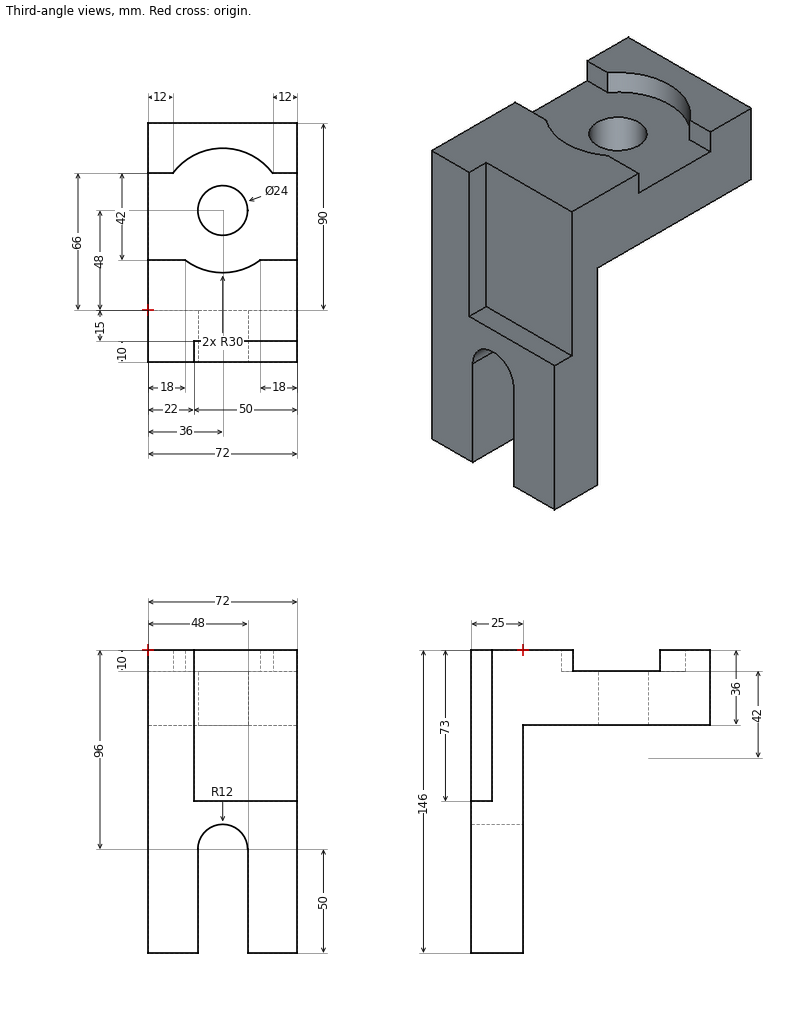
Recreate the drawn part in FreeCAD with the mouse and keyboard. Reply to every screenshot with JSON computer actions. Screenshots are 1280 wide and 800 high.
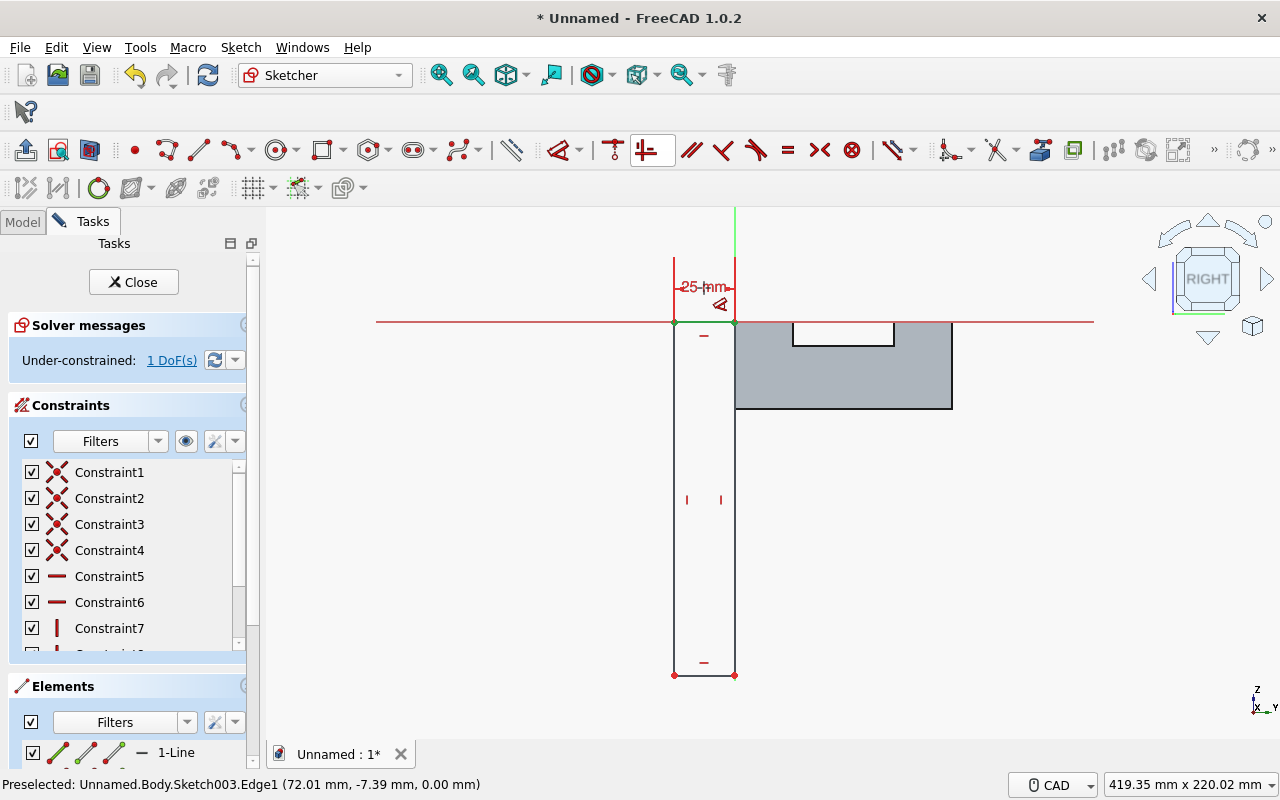
{"action": "left_click", "coordinate": [674, 428]}
{"action": "left_click", "coordinate": [640, 499]}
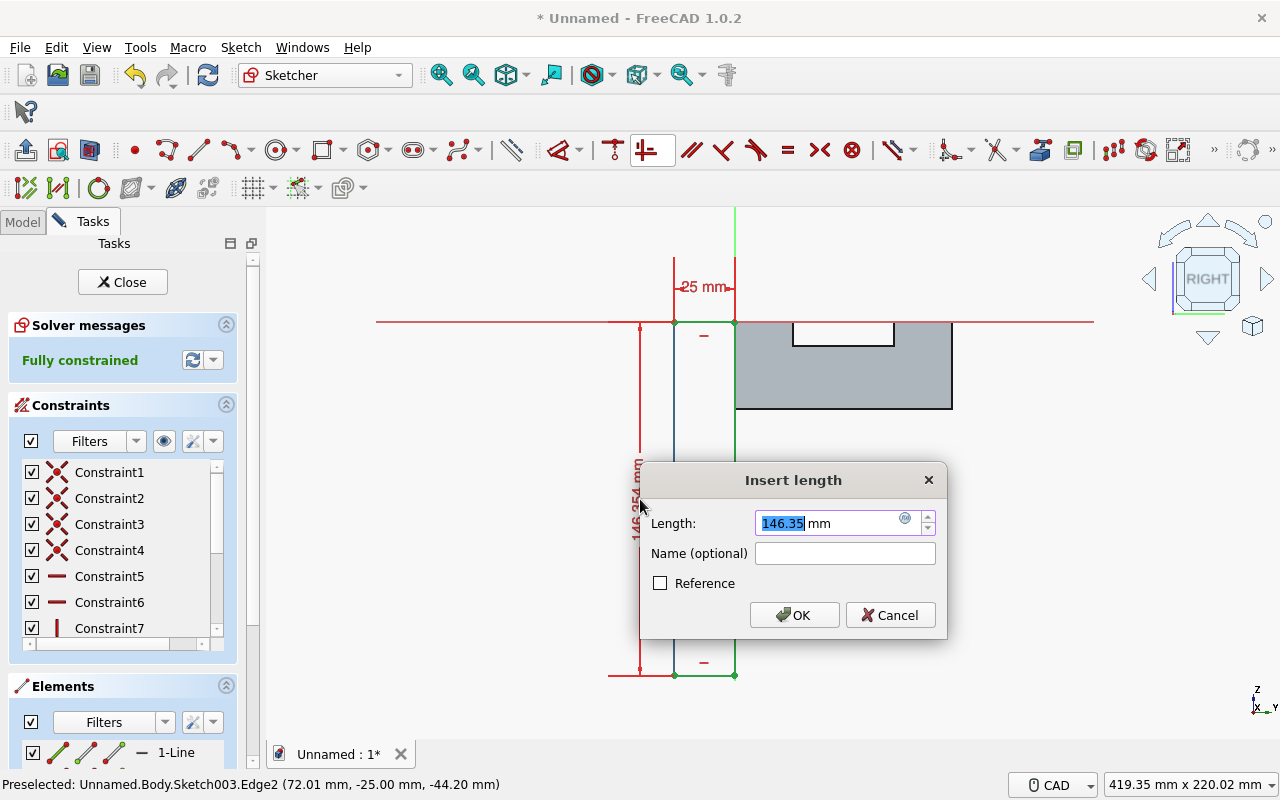
{"action": "type", "text": "146"}
{"action": "key", "text": "Return"}
{"action": "key", "text": "Escape"}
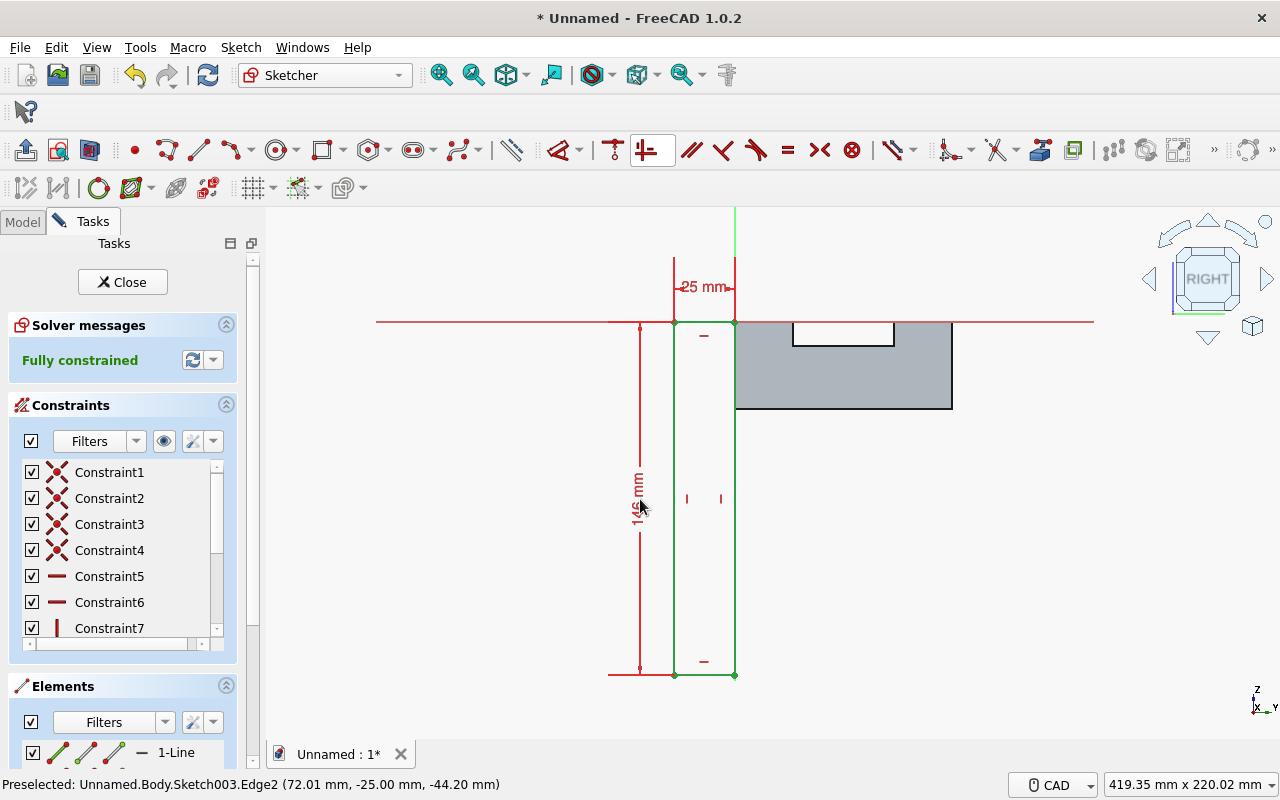
{"action": "left_click", "coordinate": [123, 282]}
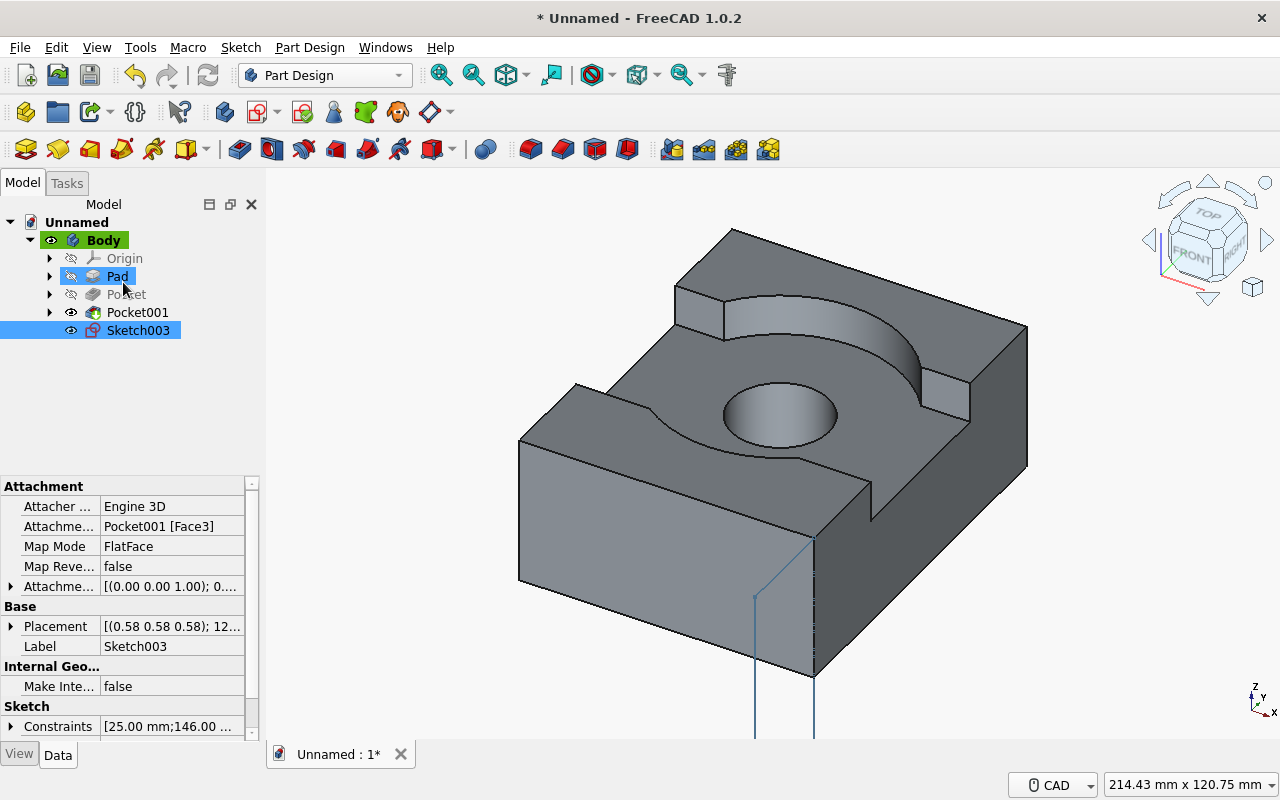
{"action": "left_click", "coordinate": [26, 150]}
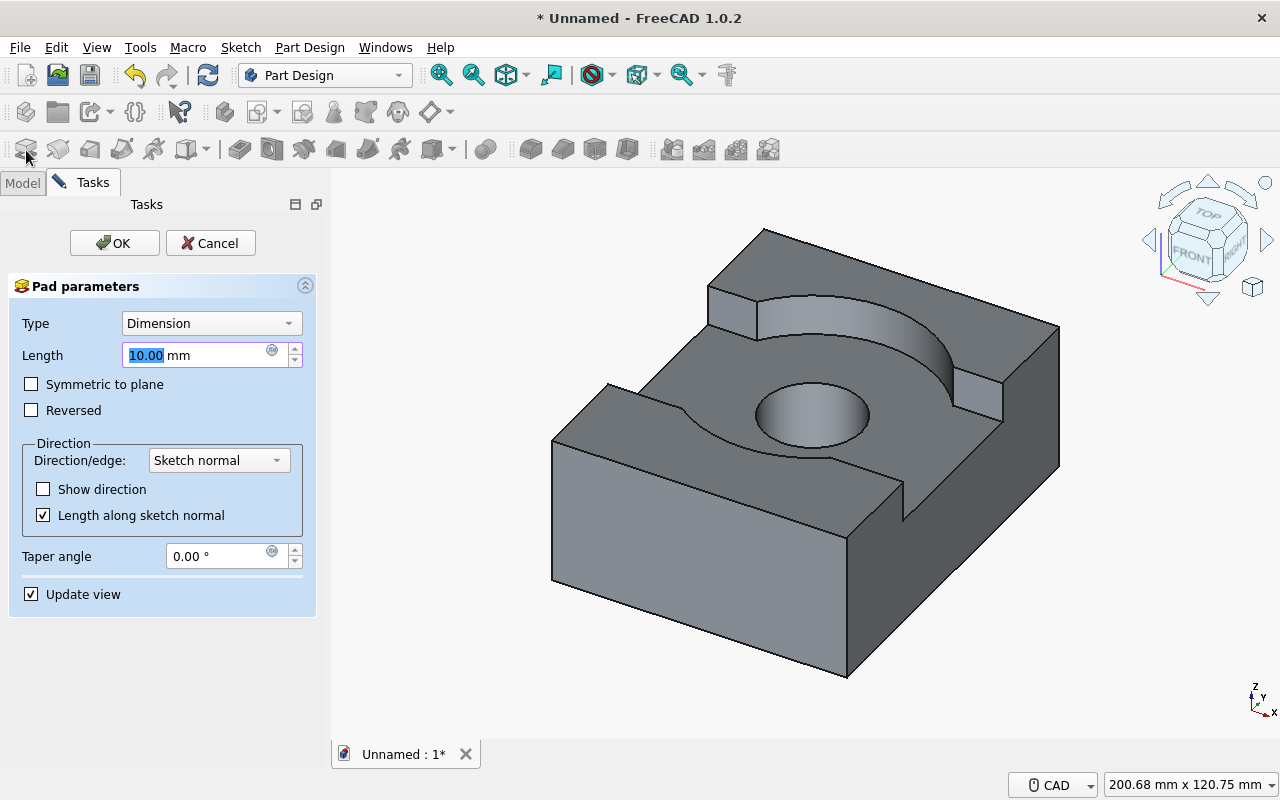
{"action": "type", "text": "72"}
{"action": "key", "text": "Tab"}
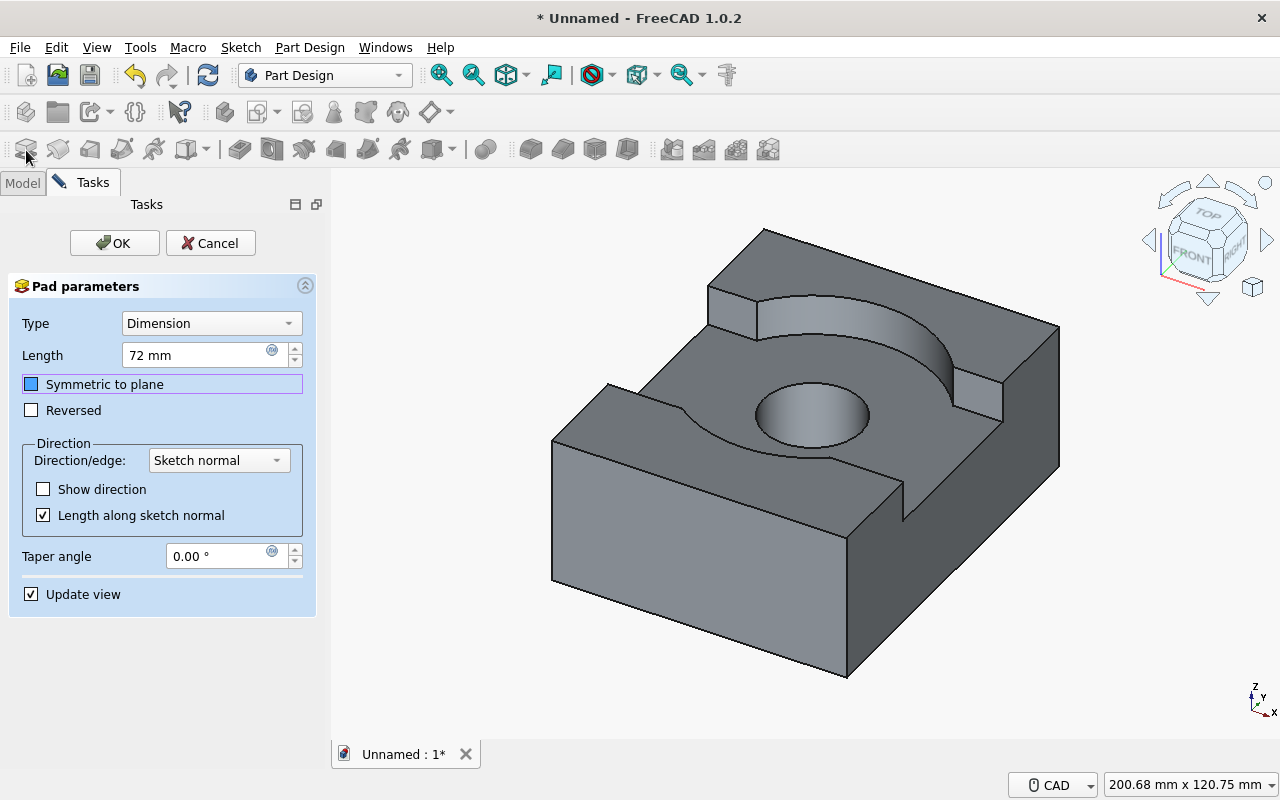
{"action": "left_click", "coordinate": [30, 410]}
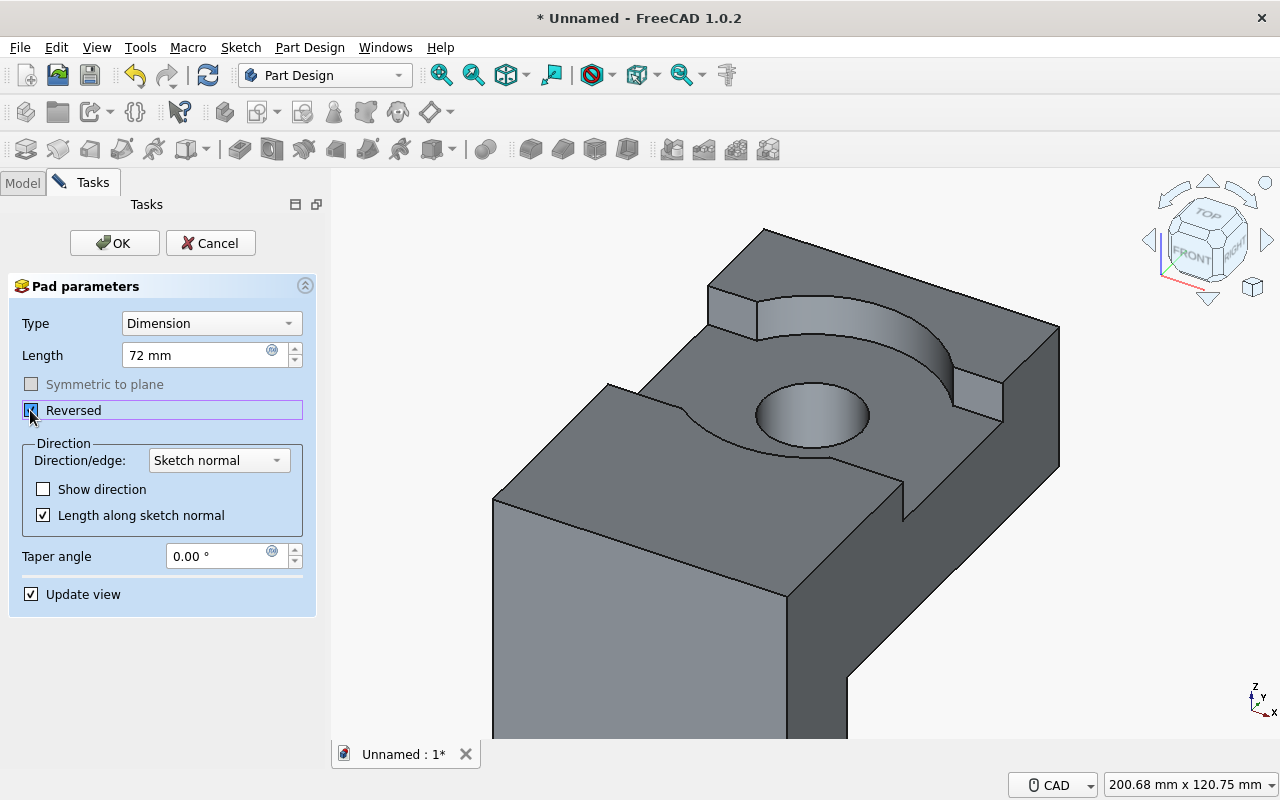
{"action": "left_click", "coordinate": [115, 243]}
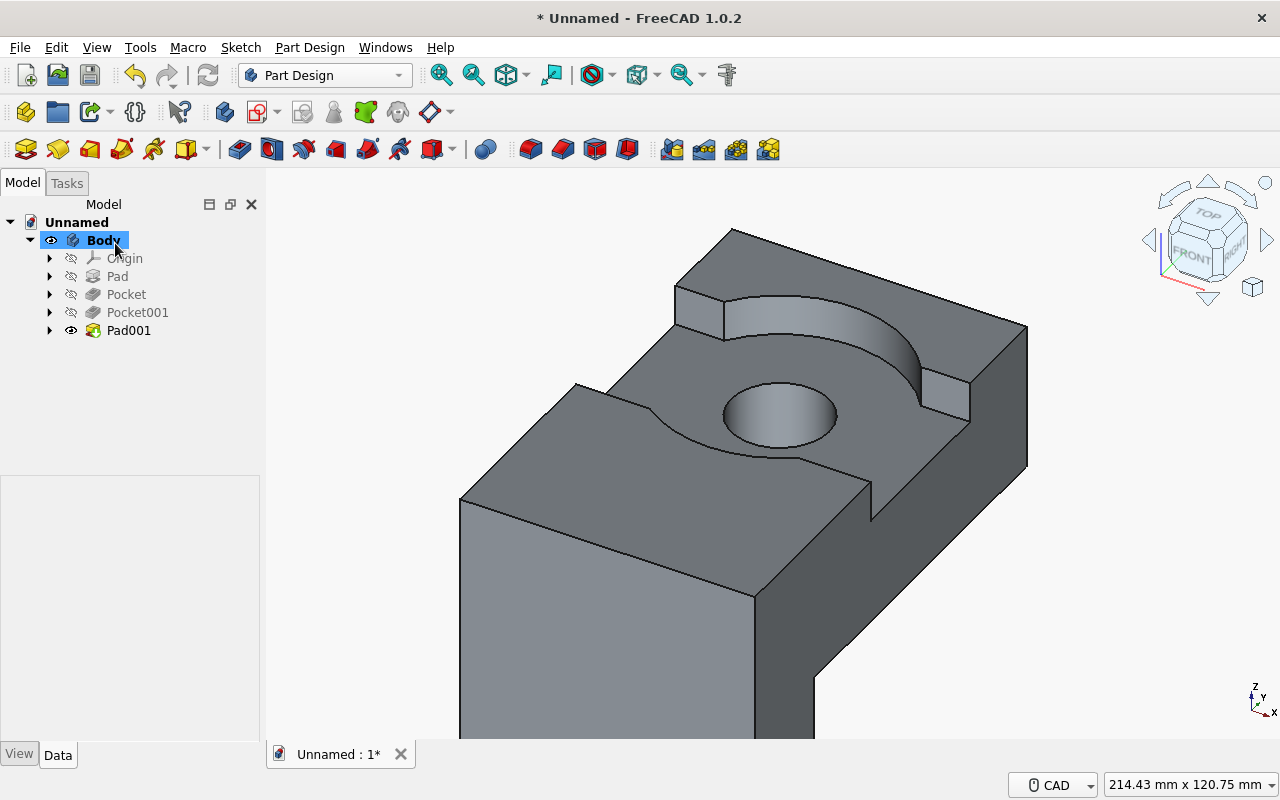
{"action": "left_click", "coordinate": [442, 76]}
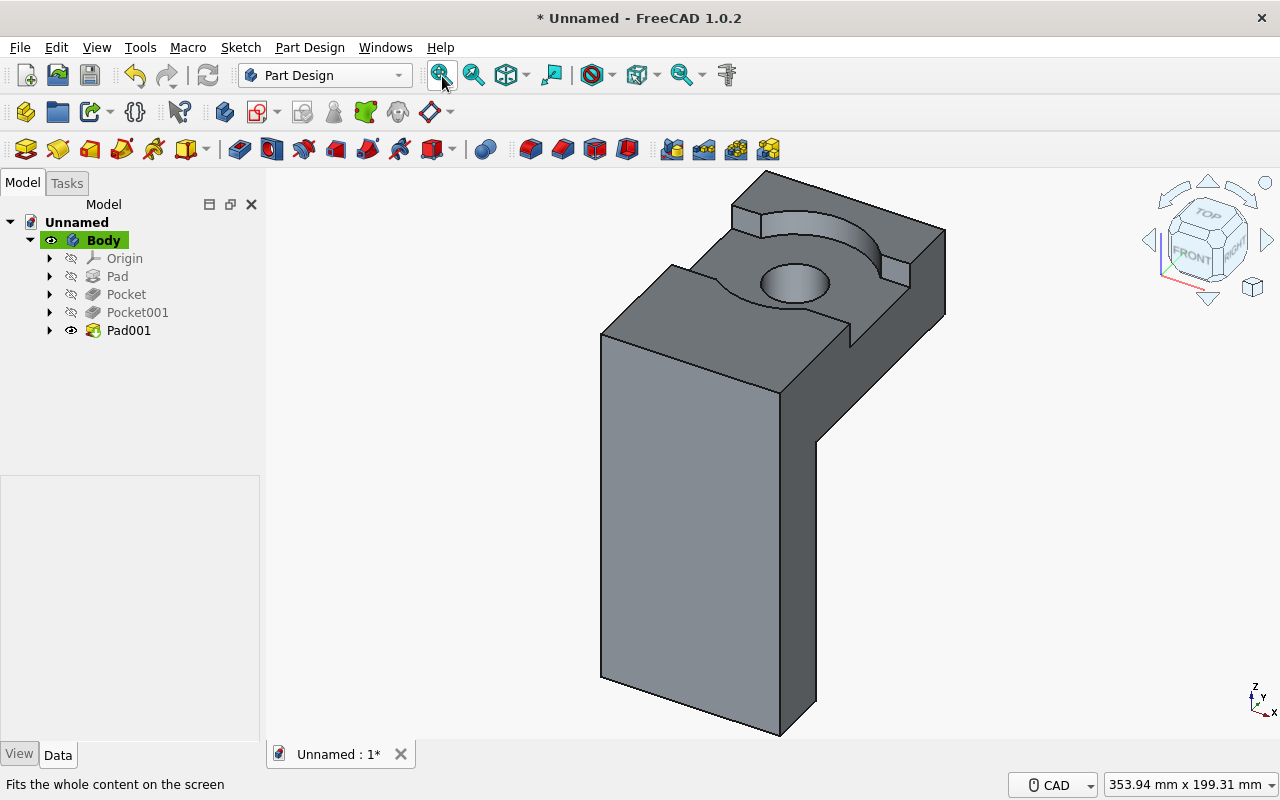
{"action": "key", "text": "4"}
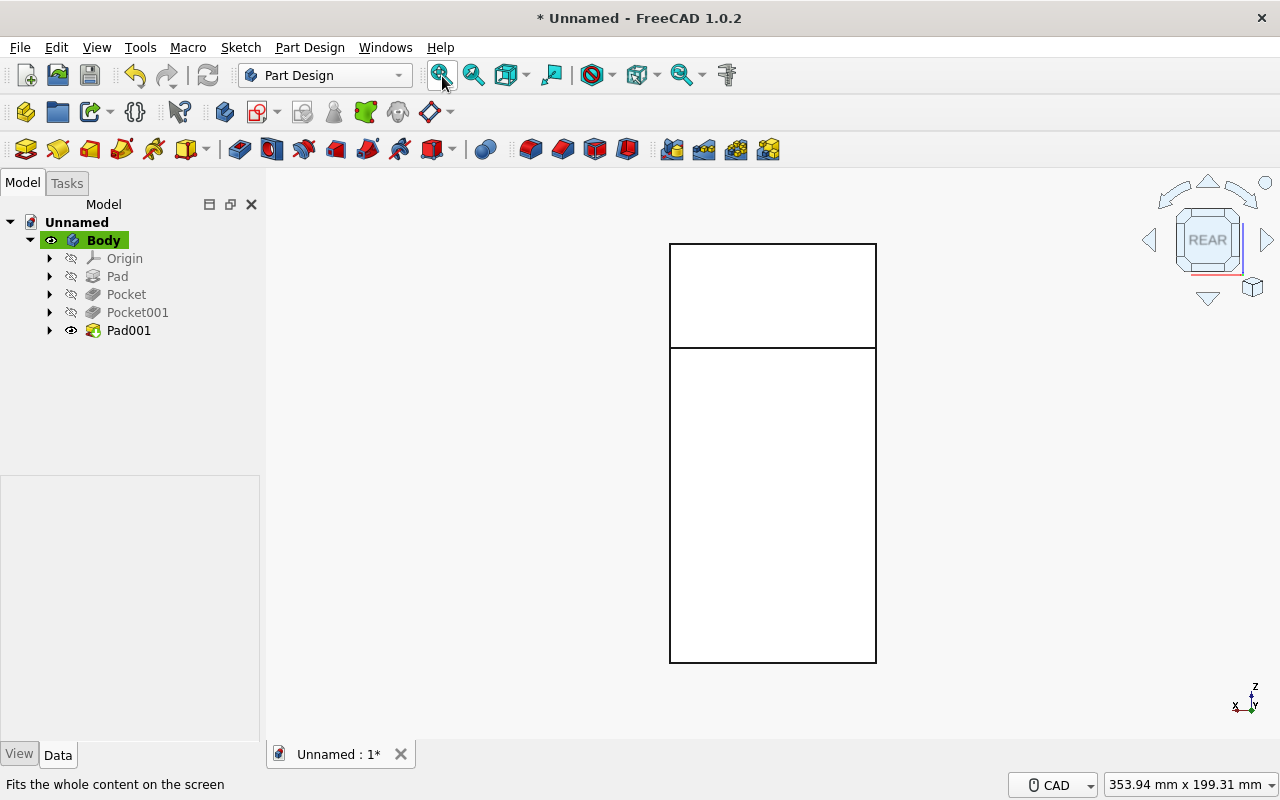
{"action": "left_click", "coordinate": [773, 459]}